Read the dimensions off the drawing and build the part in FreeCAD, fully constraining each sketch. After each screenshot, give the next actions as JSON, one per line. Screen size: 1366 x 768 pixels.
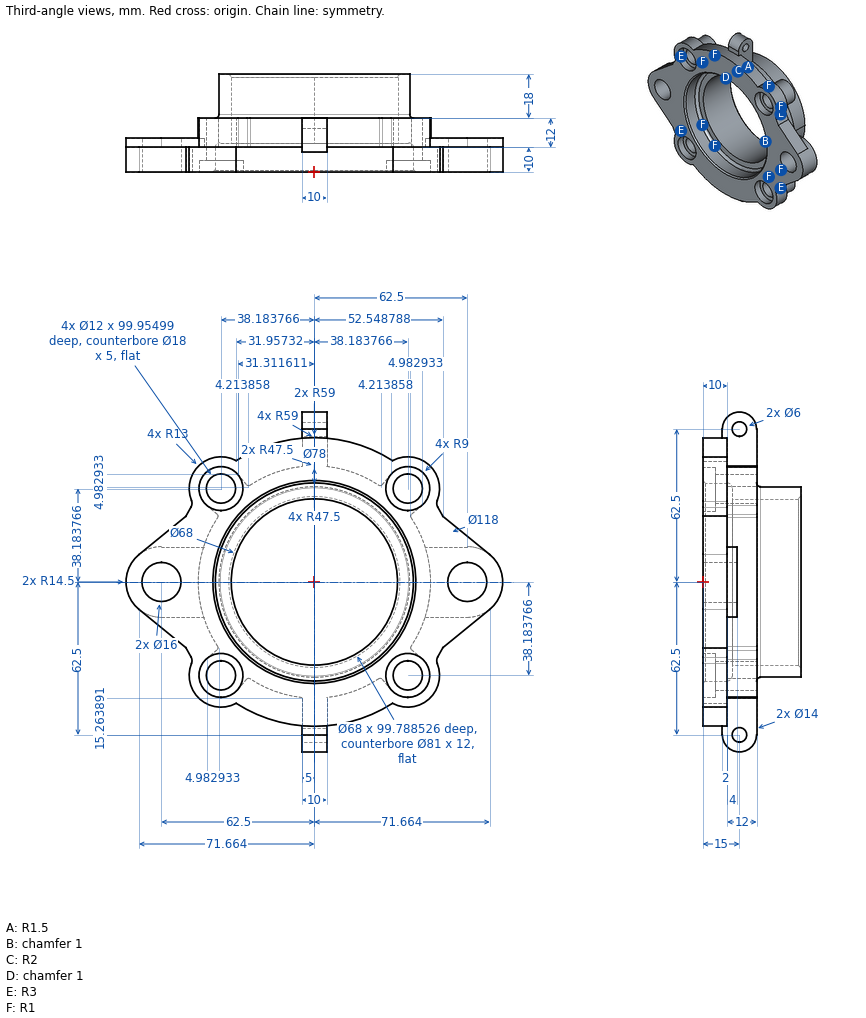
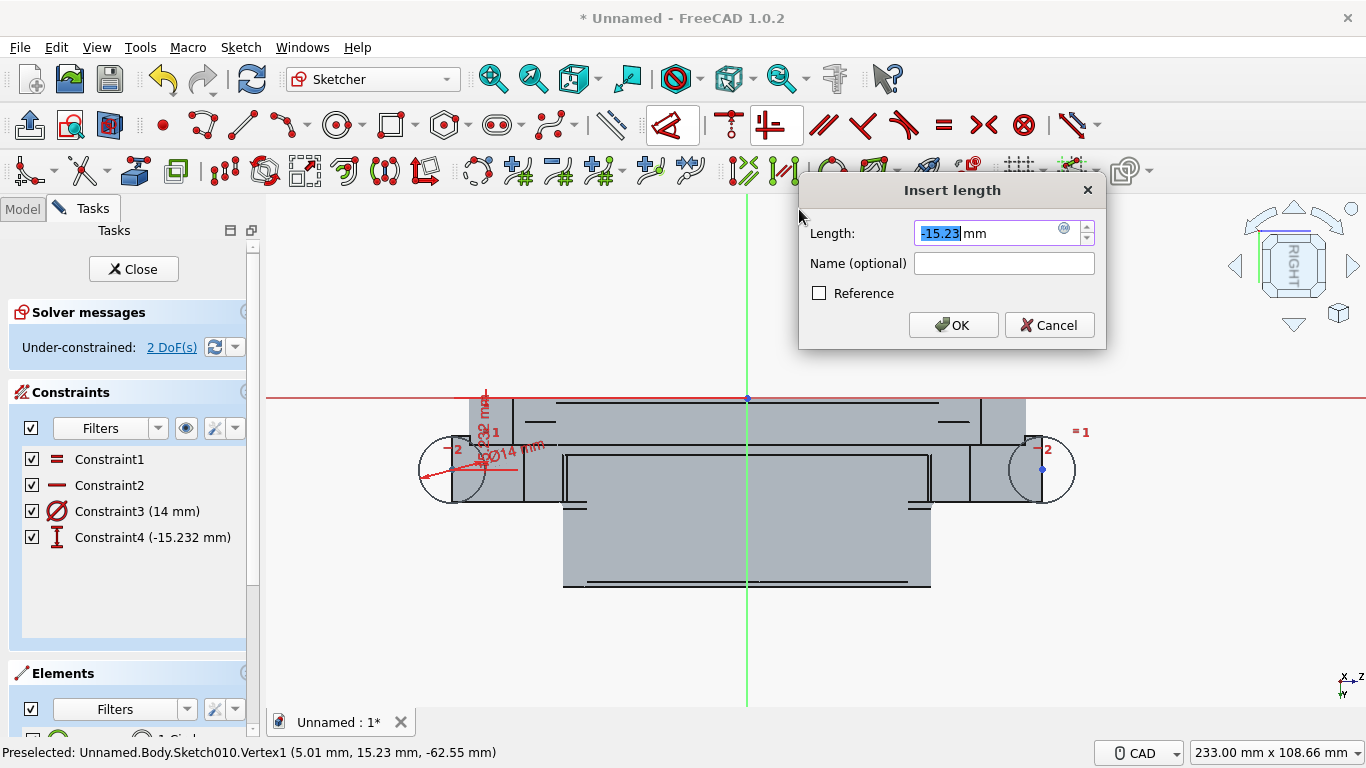
{"action": "type", "text": "-15"}
{"action": "key", "text": "Return"}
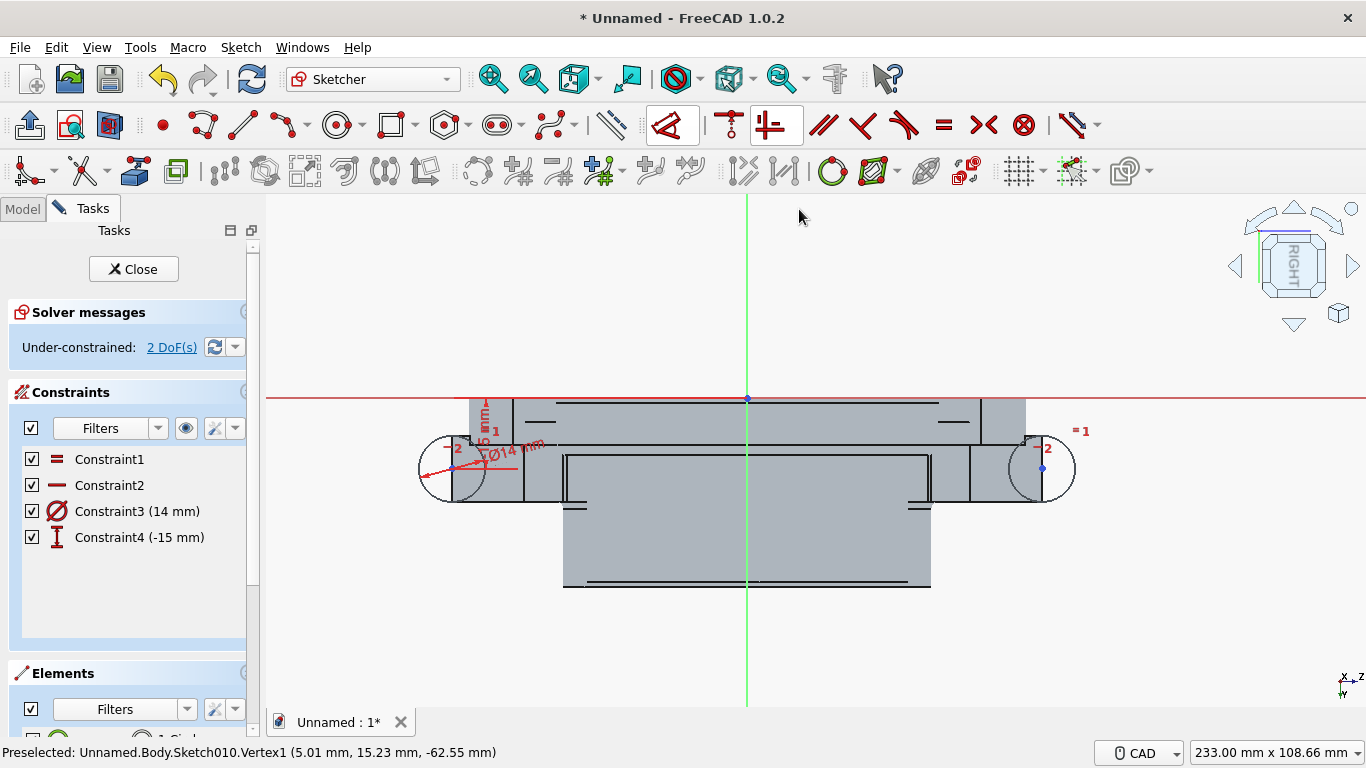
{"action": "left_click", "coordinate": [452, 469]}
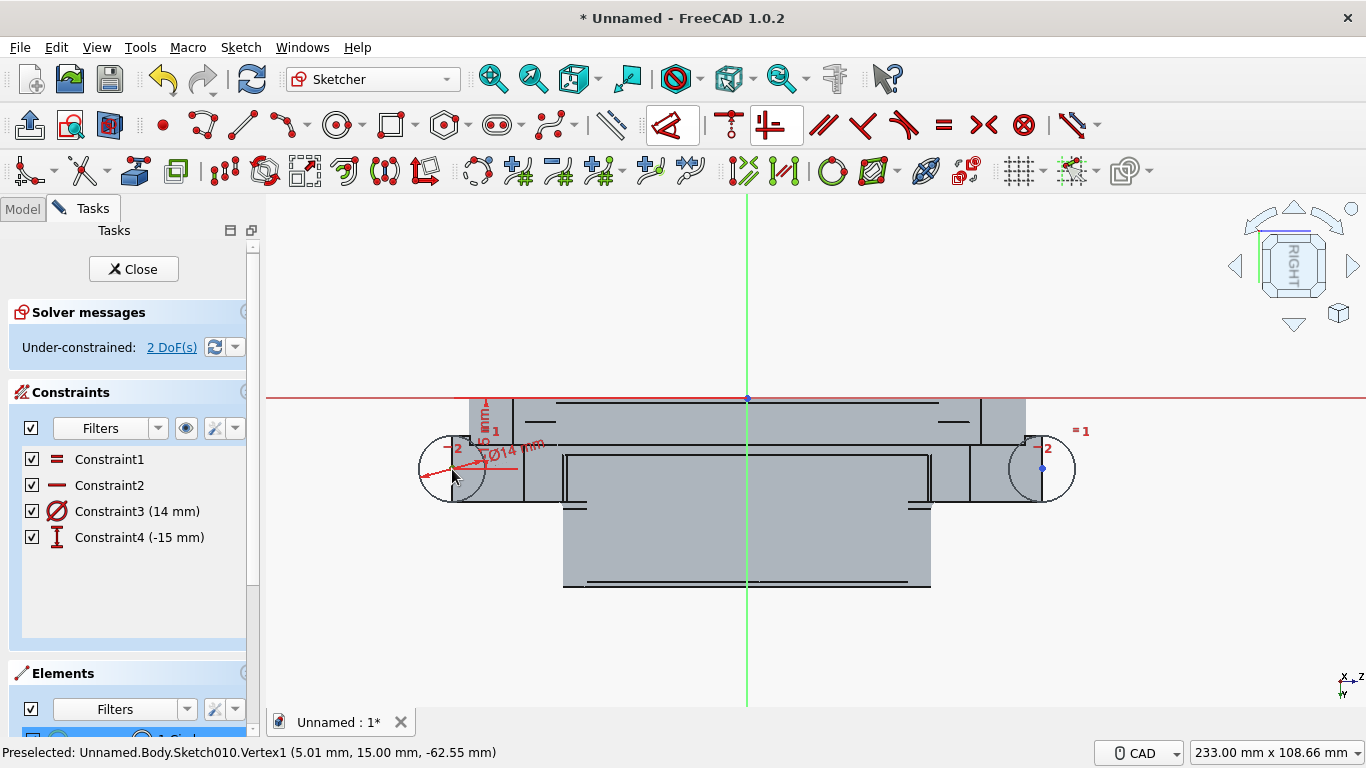
{"action": "left_click", "coordinate": [694, 126]}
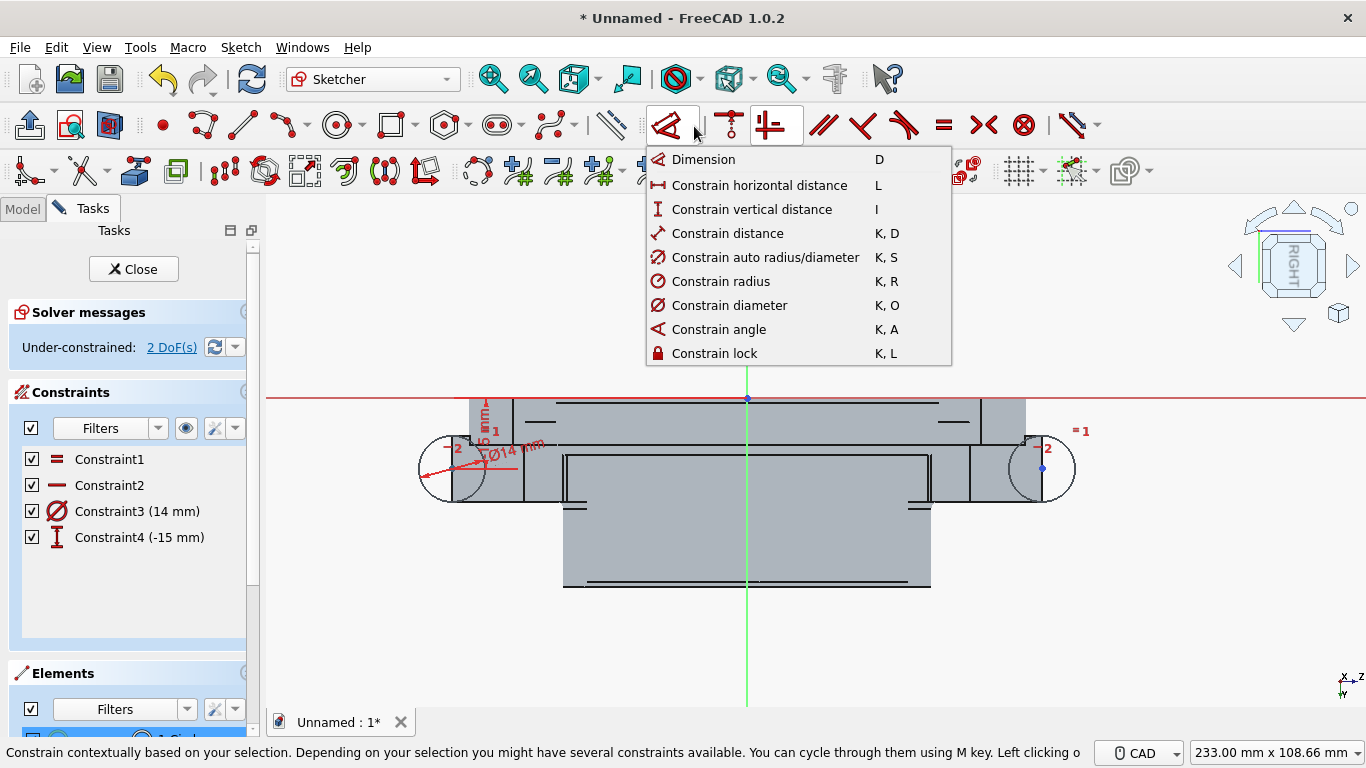
{"action": "left_click", "coordinate": [799, 185]}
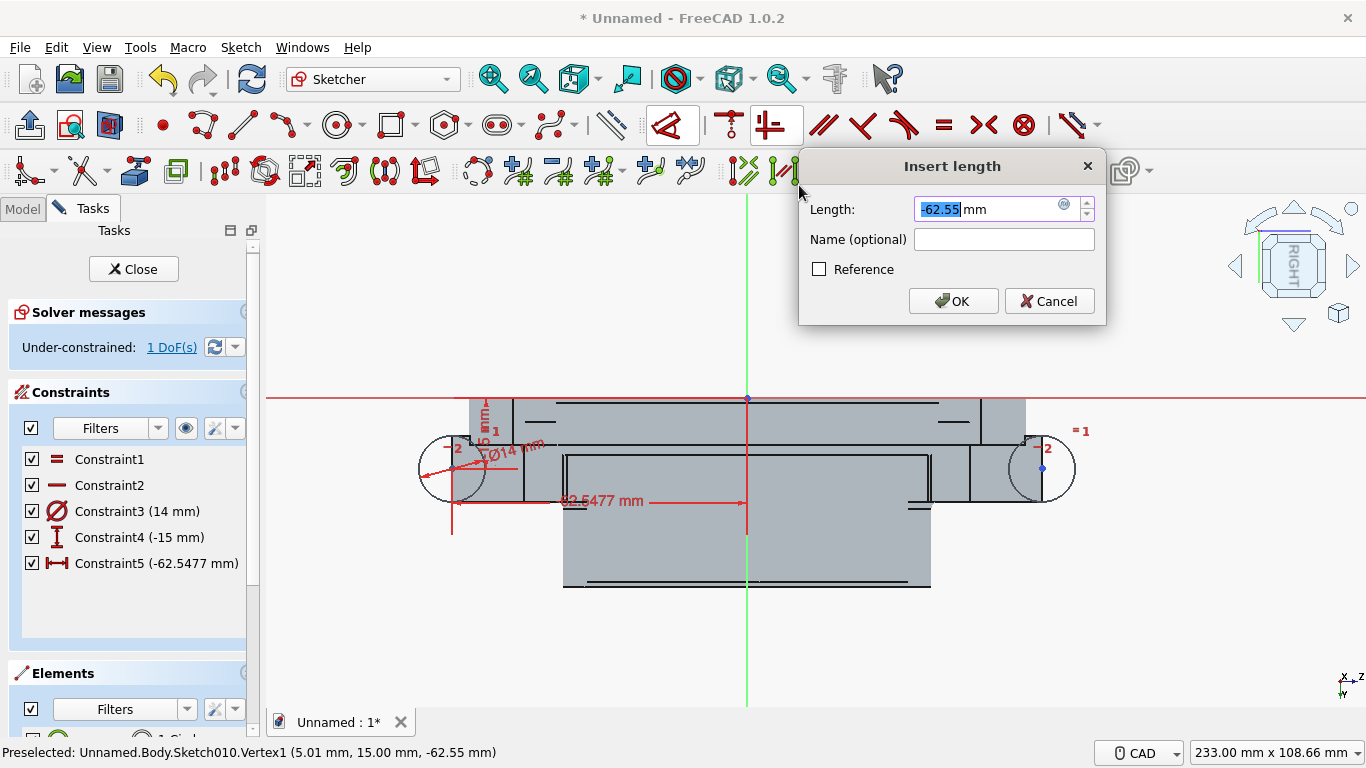
{"action": "type", "text": "-62.5"}
{"action": "key", "text": "Return"}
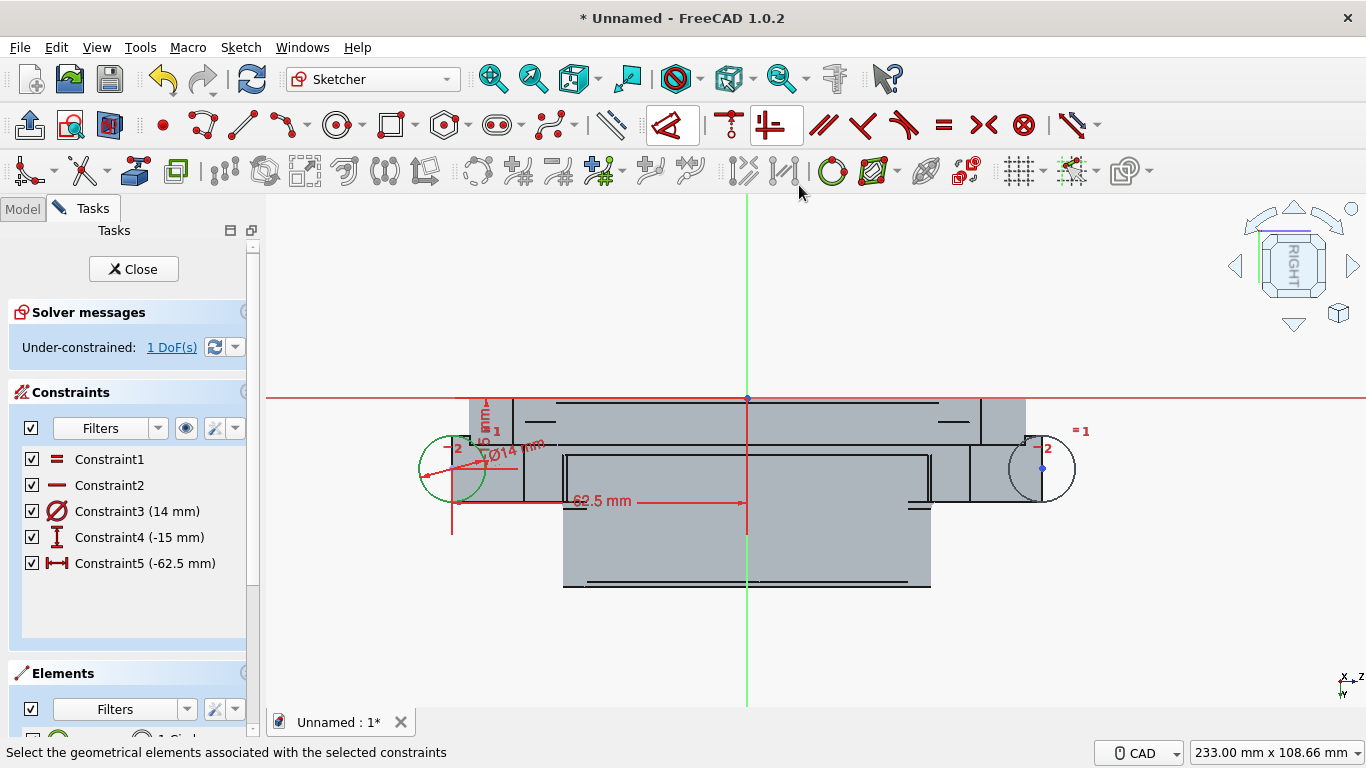
{"action": "left_click", "coordinate": [1042, 469]}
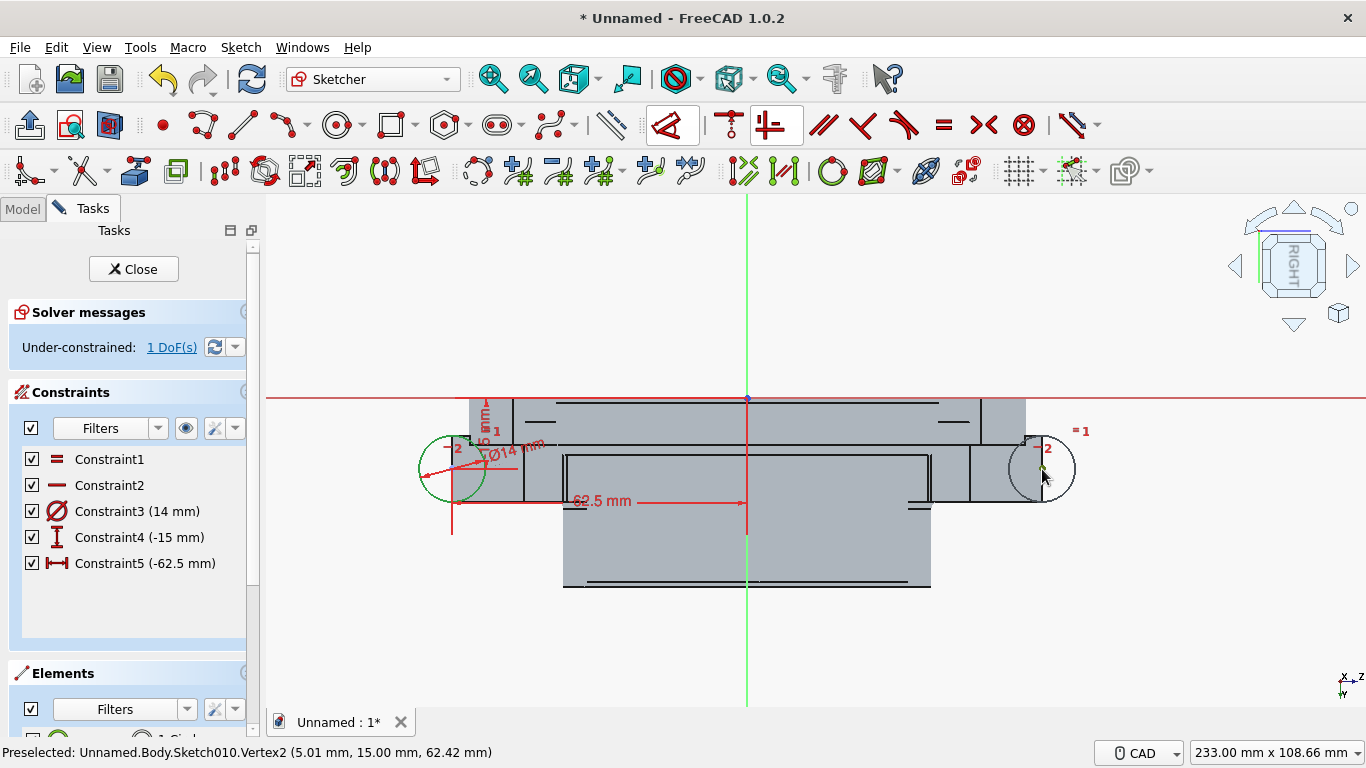
{"action": "left_click", "coordinate": [694, 126]}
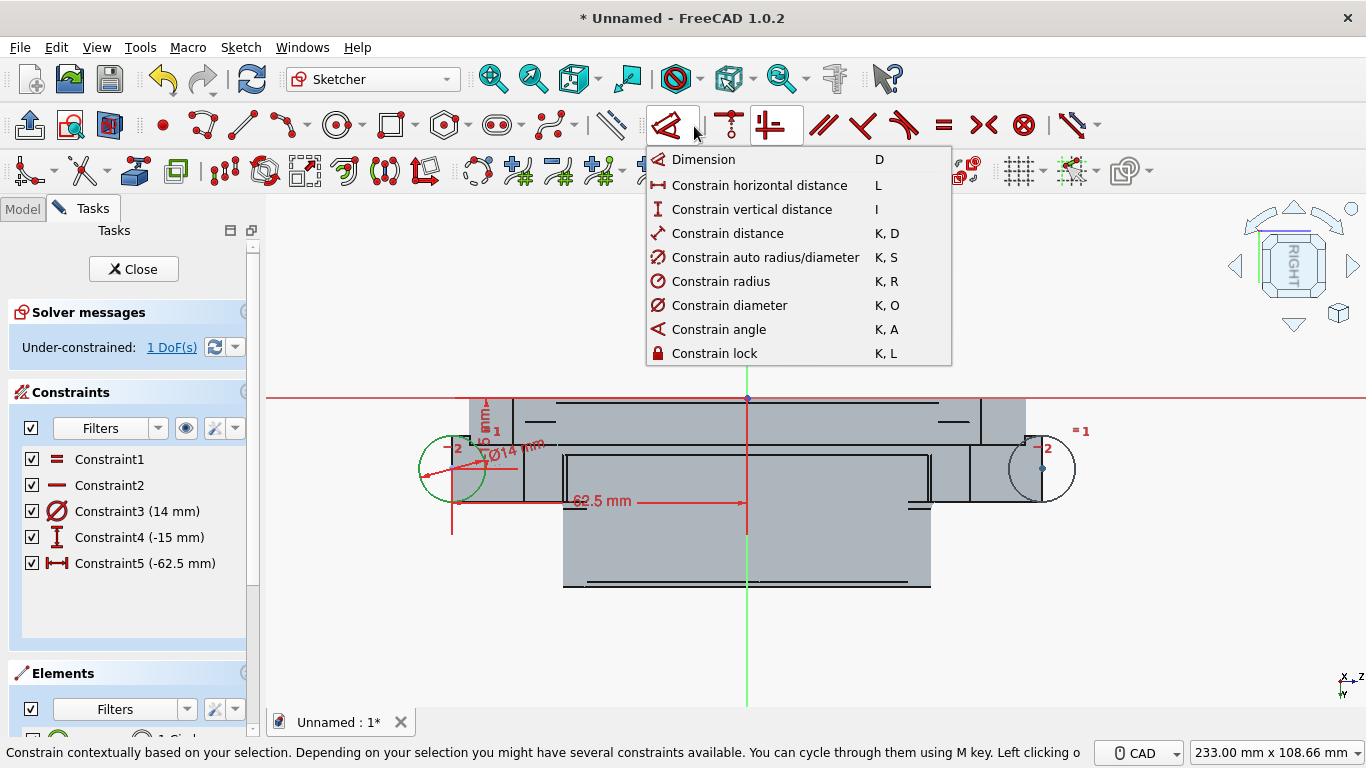
{"action": "left_click", "coordinate": [799, 185]}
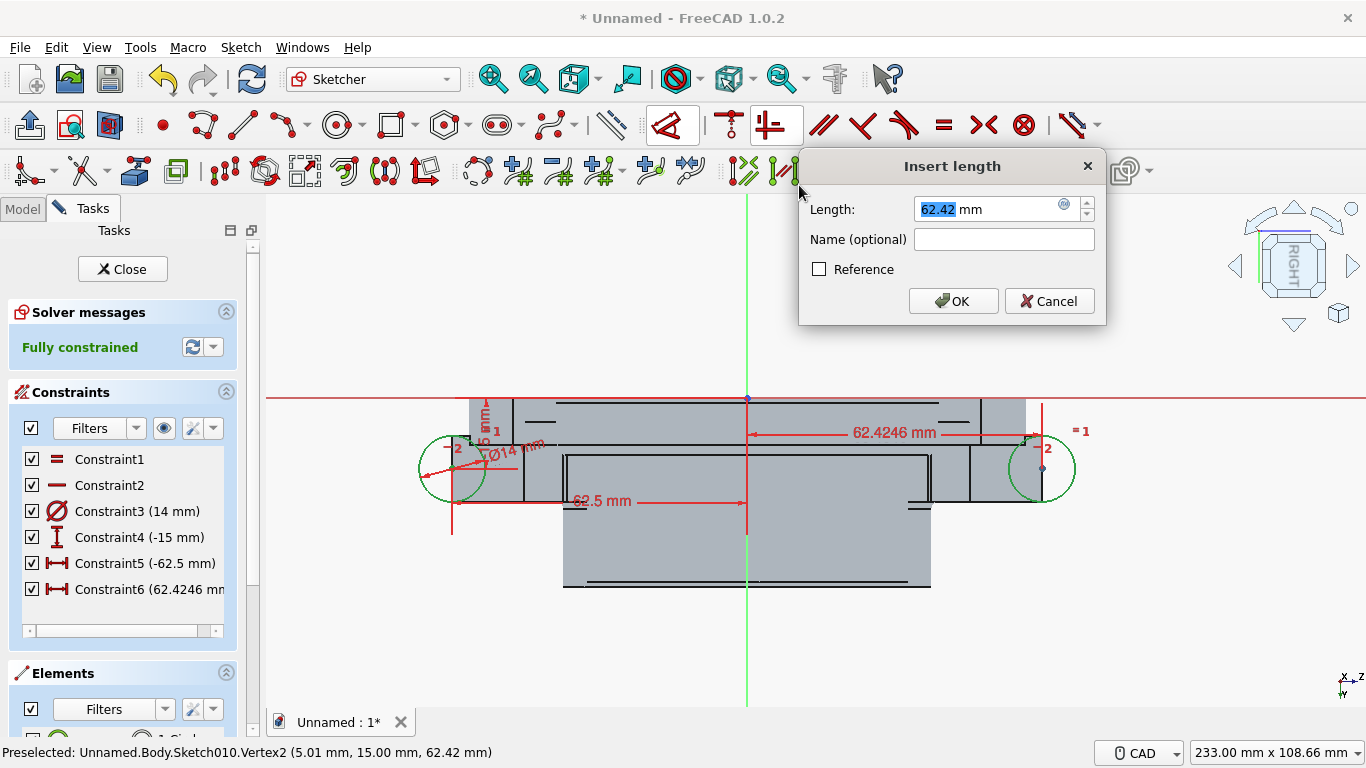
{"action": "type", "text": "62.5"}
{"action": "key", "text": "Return"}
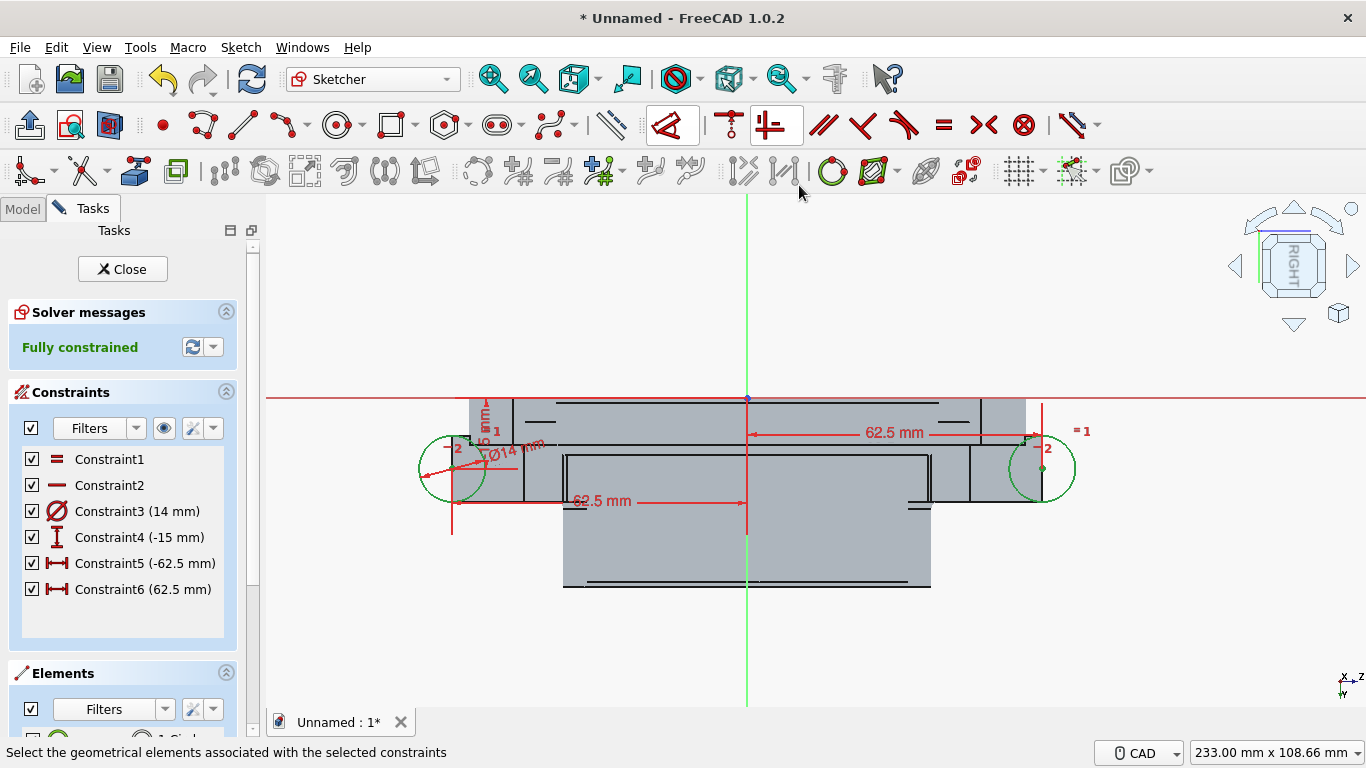
{"action": "left_click", "coordinate": [123, 269]}